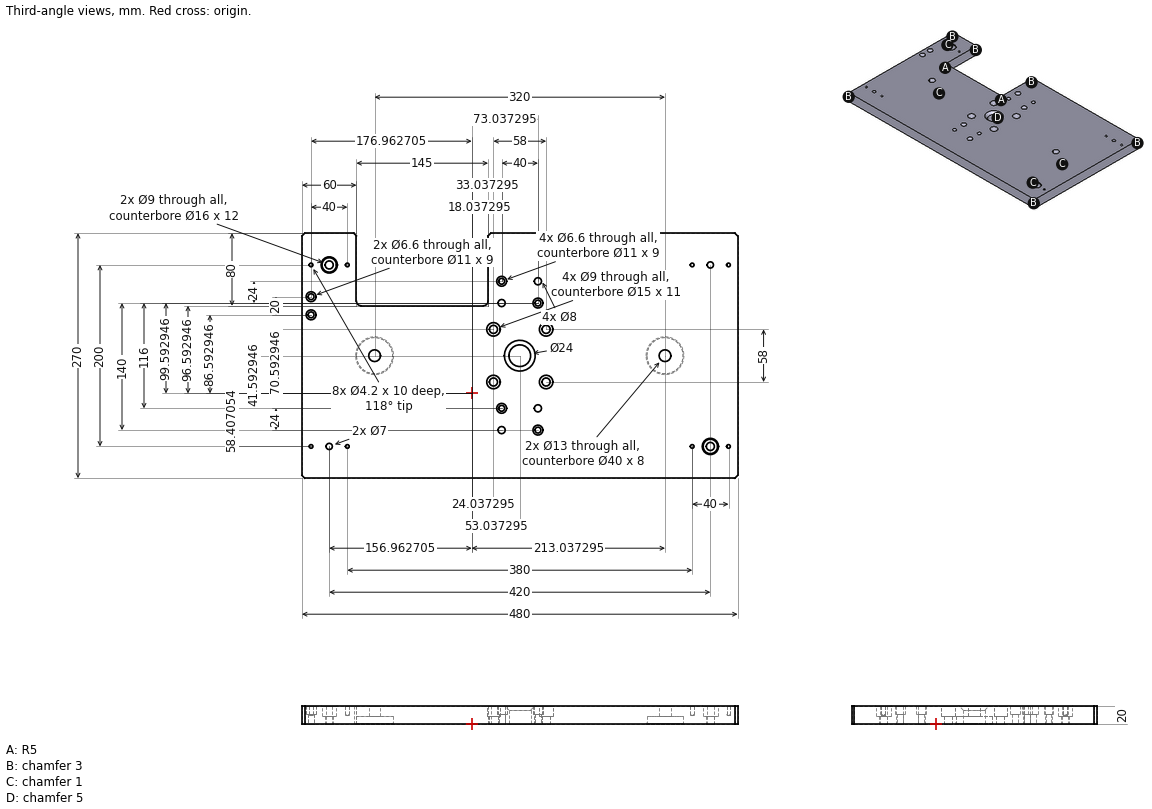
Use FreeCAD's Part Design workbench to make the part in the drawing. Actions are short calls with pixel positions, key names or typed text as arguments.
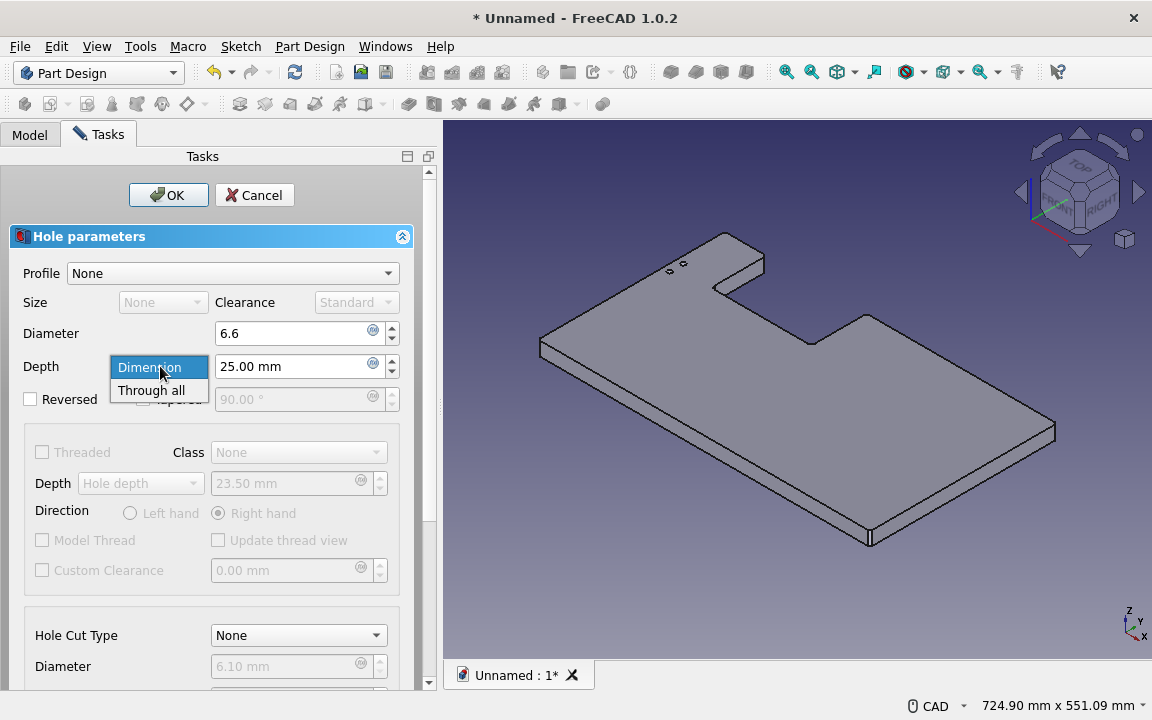
click(158, 390)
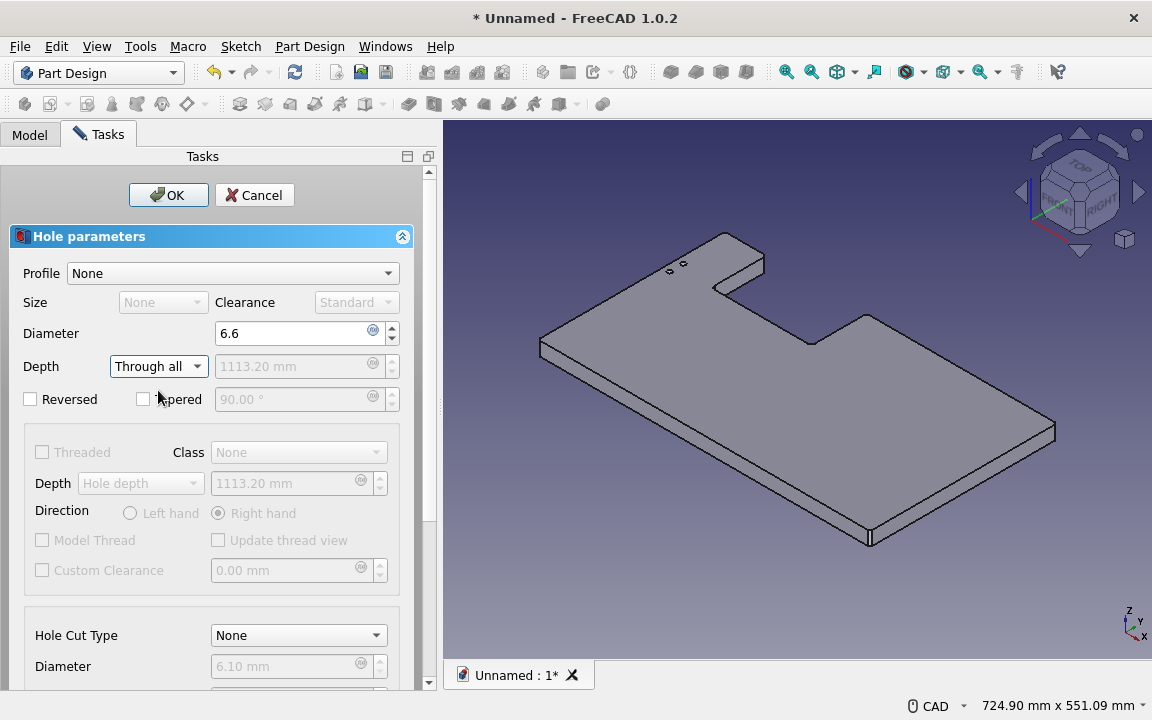
click(300, 636)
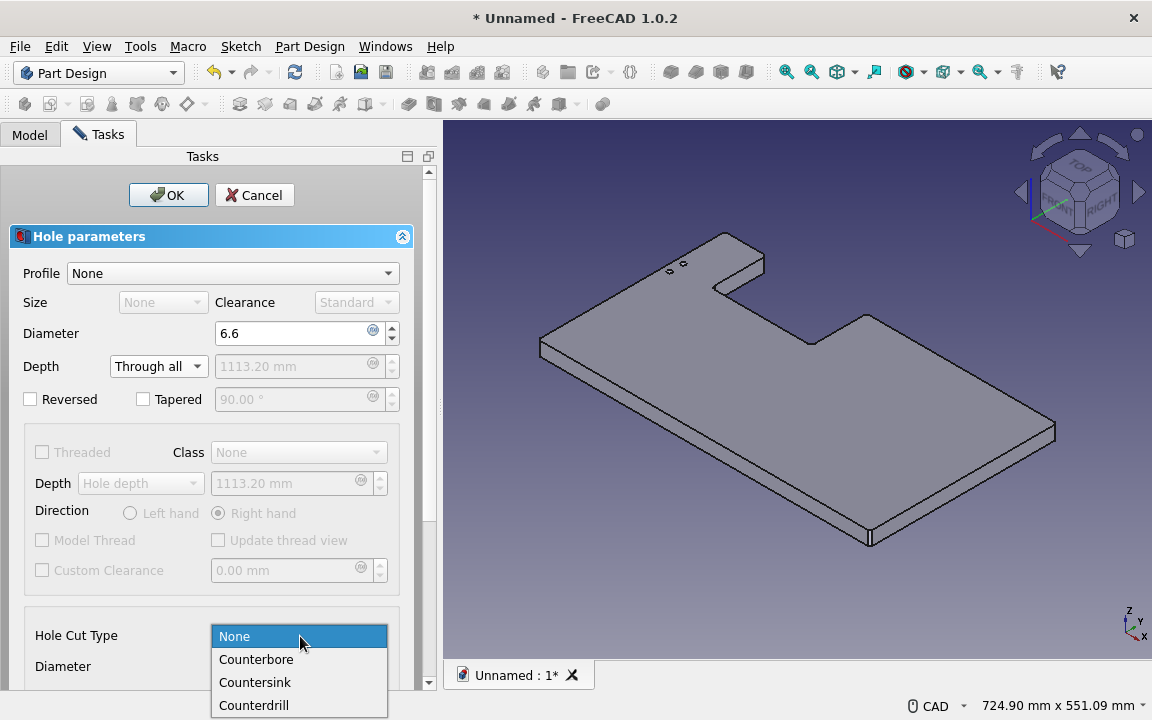
click(298, 660)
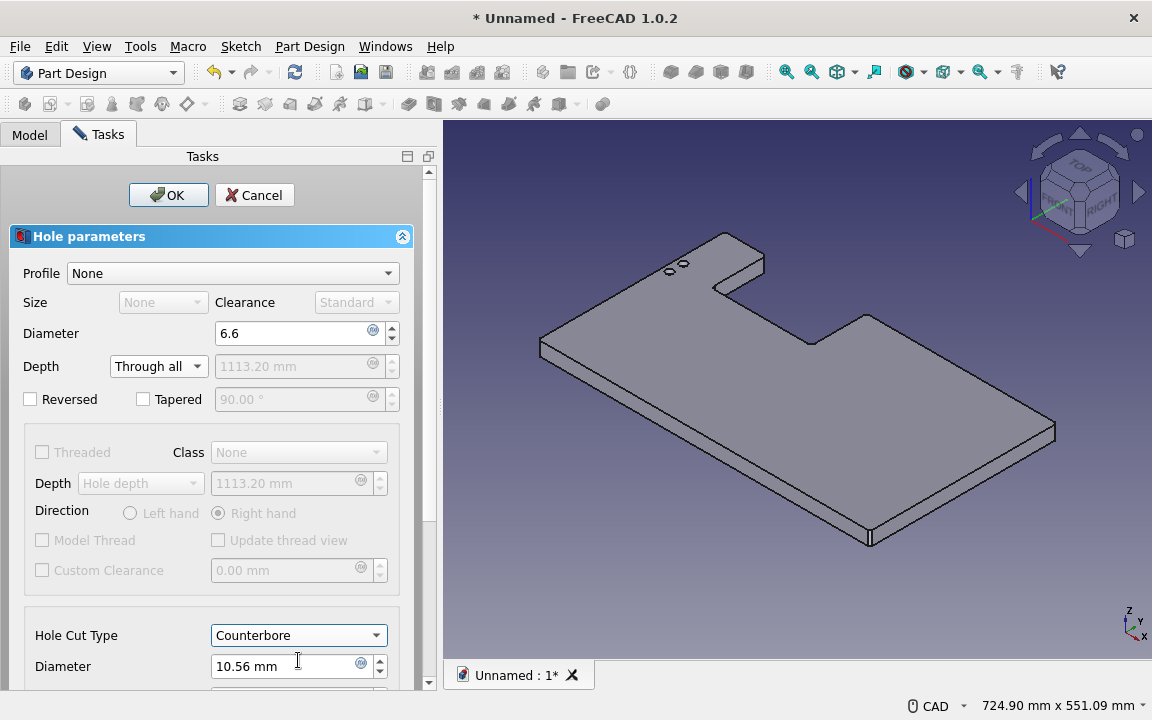
triple_click(292, 666)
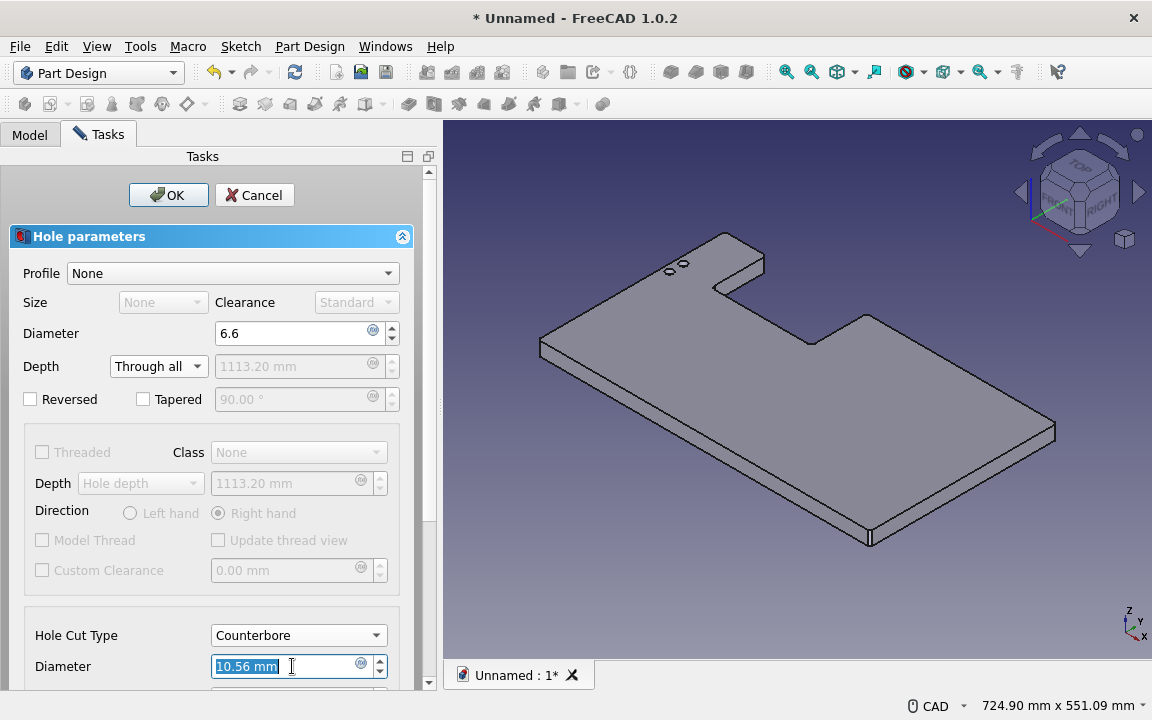
text(11)
key(Tab)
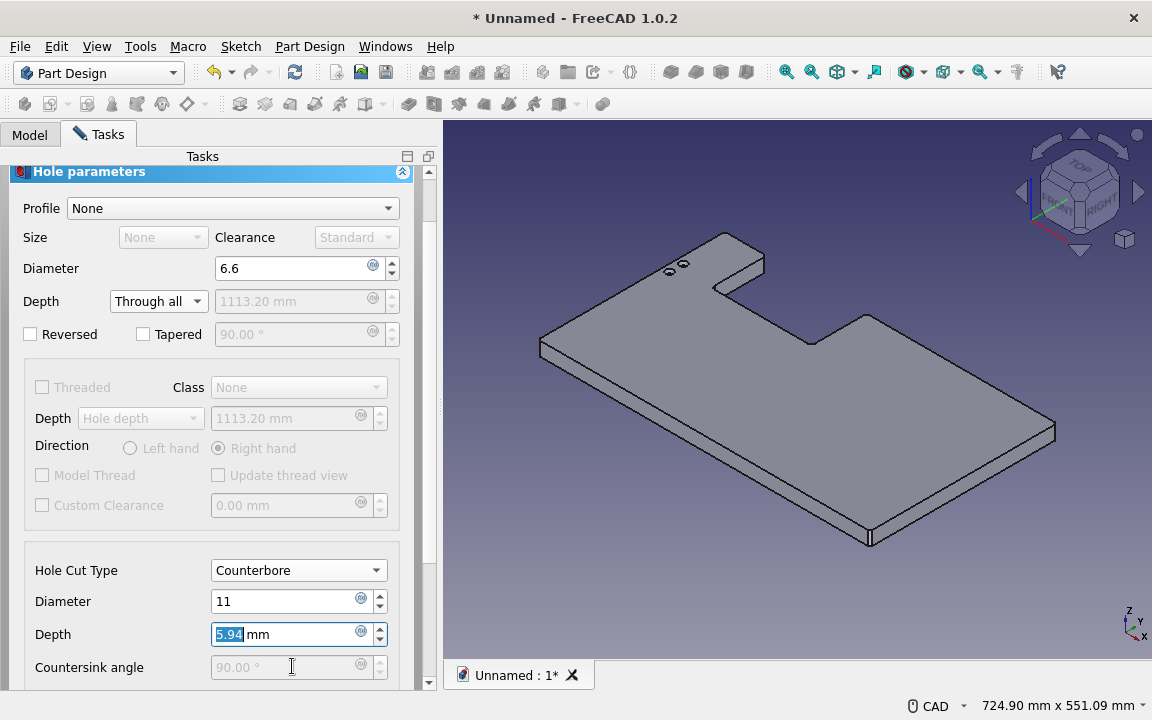
text(9)
key(Tab)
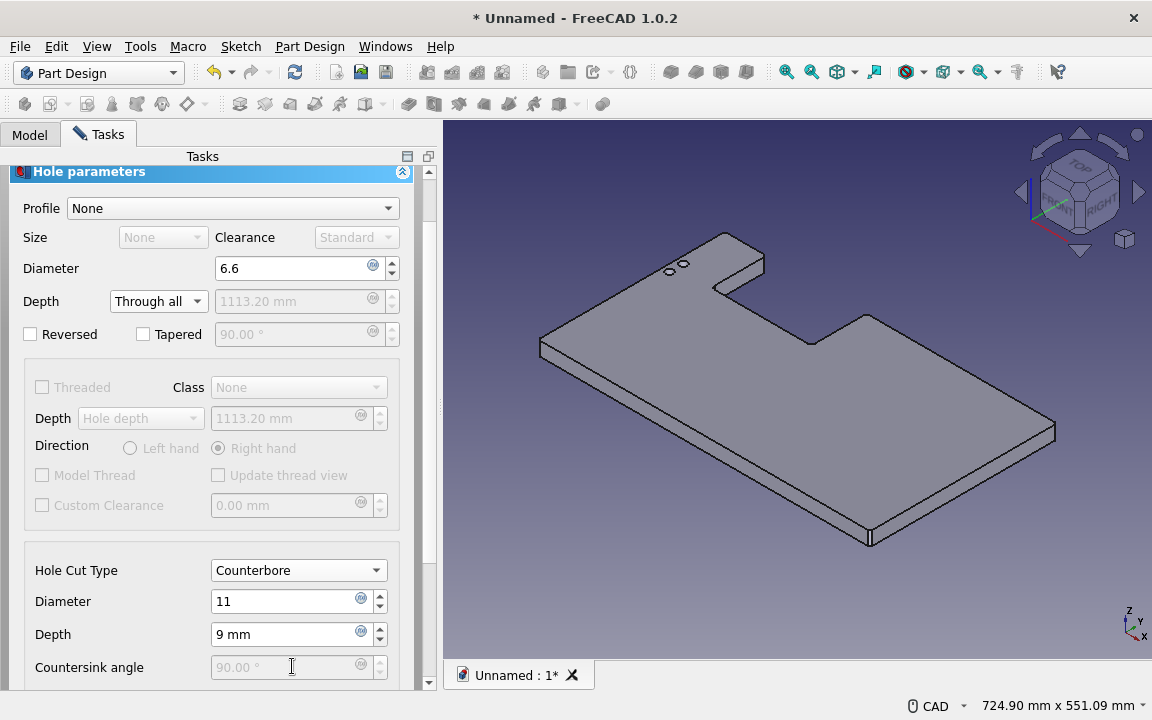
scroll(429, 428, up, 2)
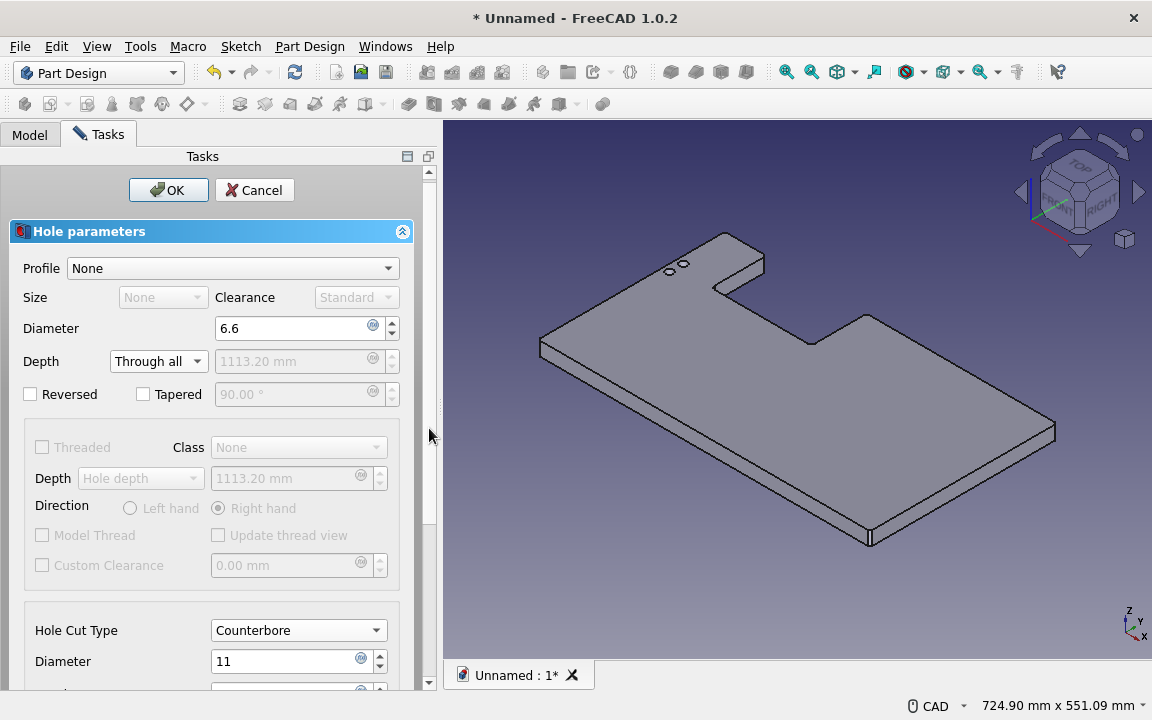
click(169, 195)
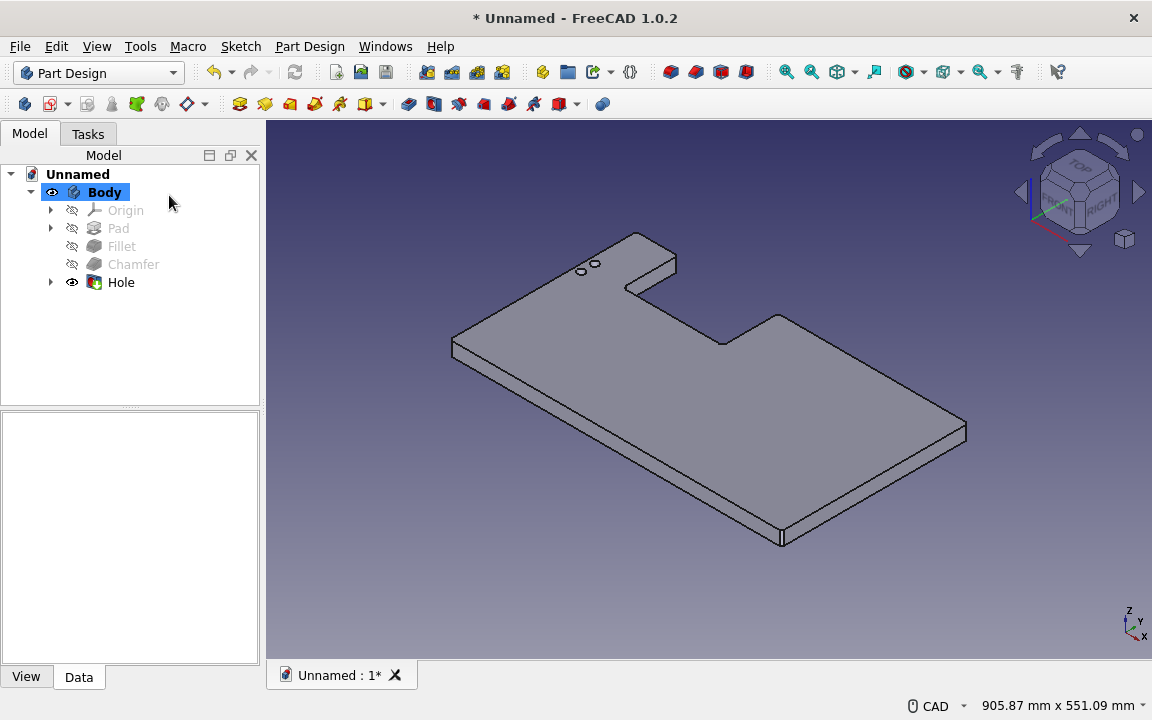
click(756, 408)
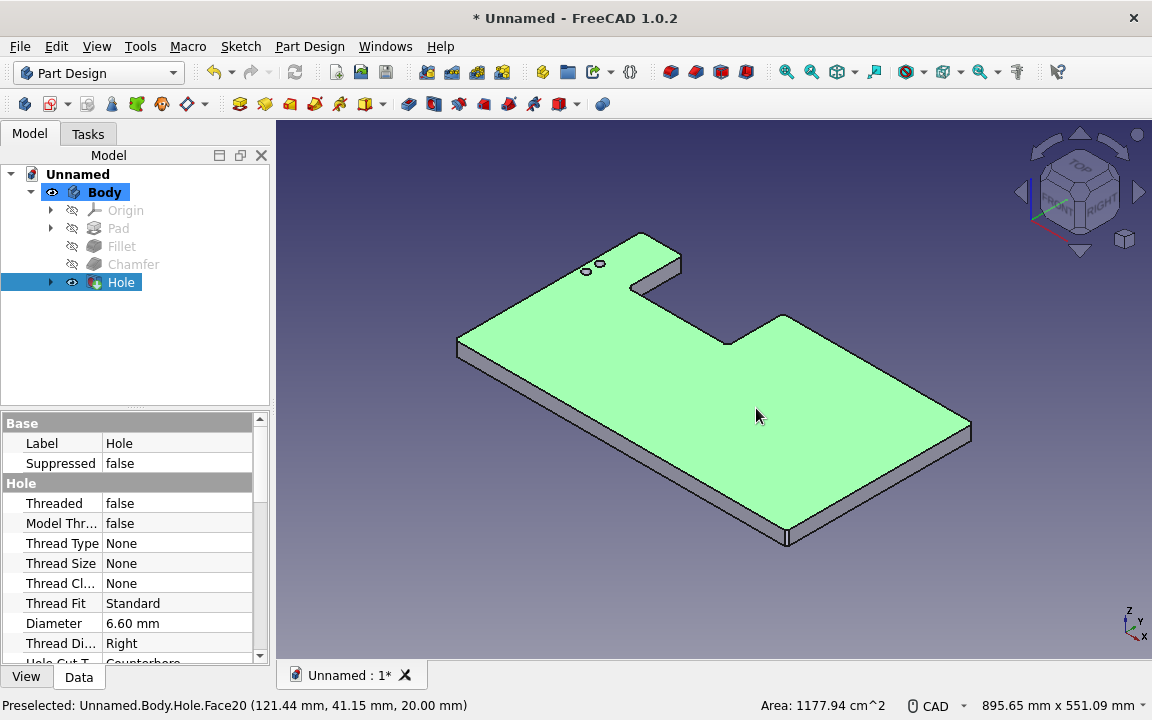
click(50, 104)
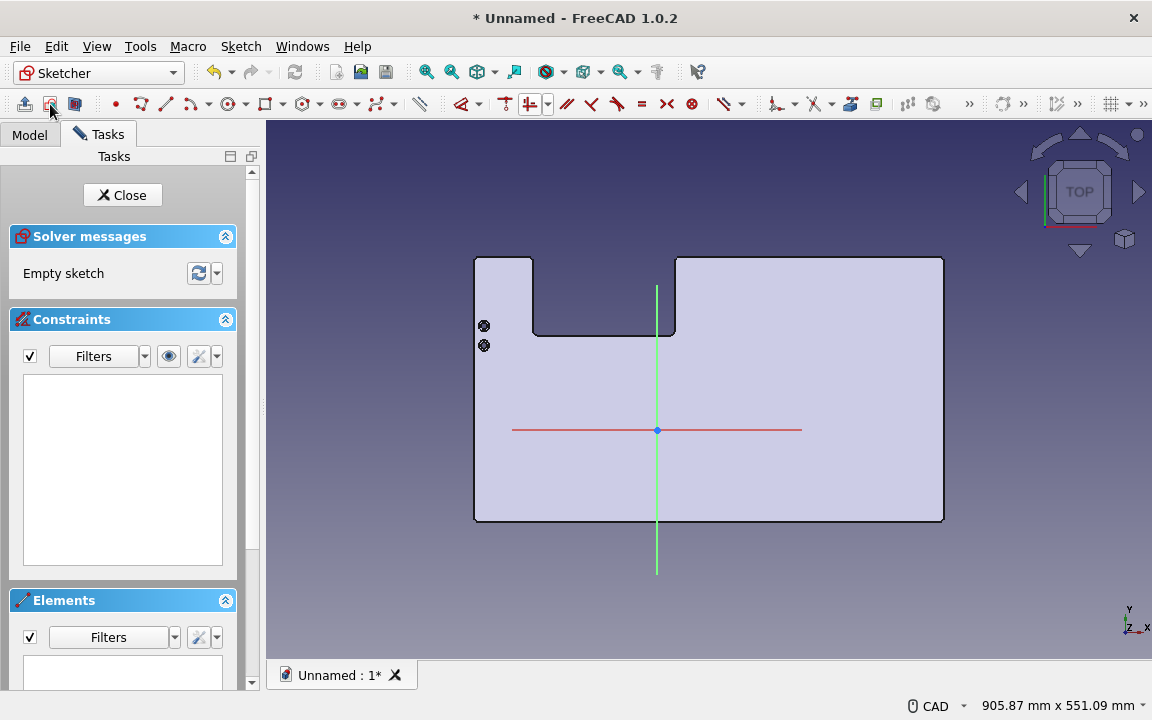
key(g)
key(c)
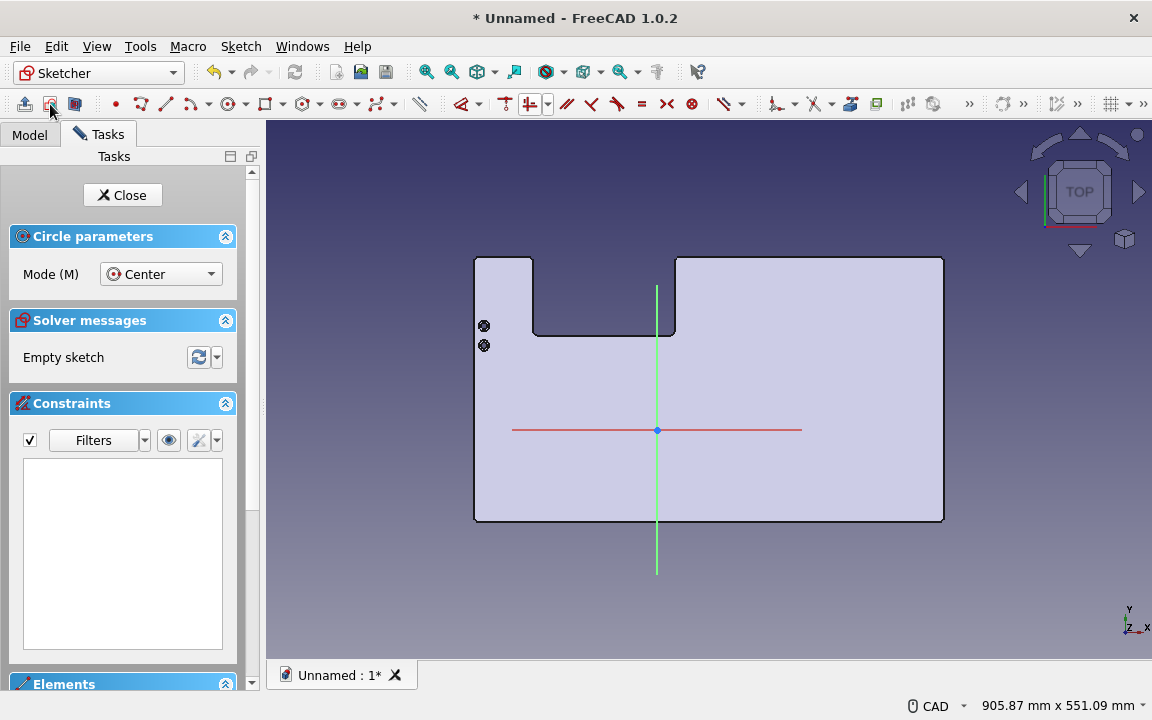
scroll(484, 292, up, 13)